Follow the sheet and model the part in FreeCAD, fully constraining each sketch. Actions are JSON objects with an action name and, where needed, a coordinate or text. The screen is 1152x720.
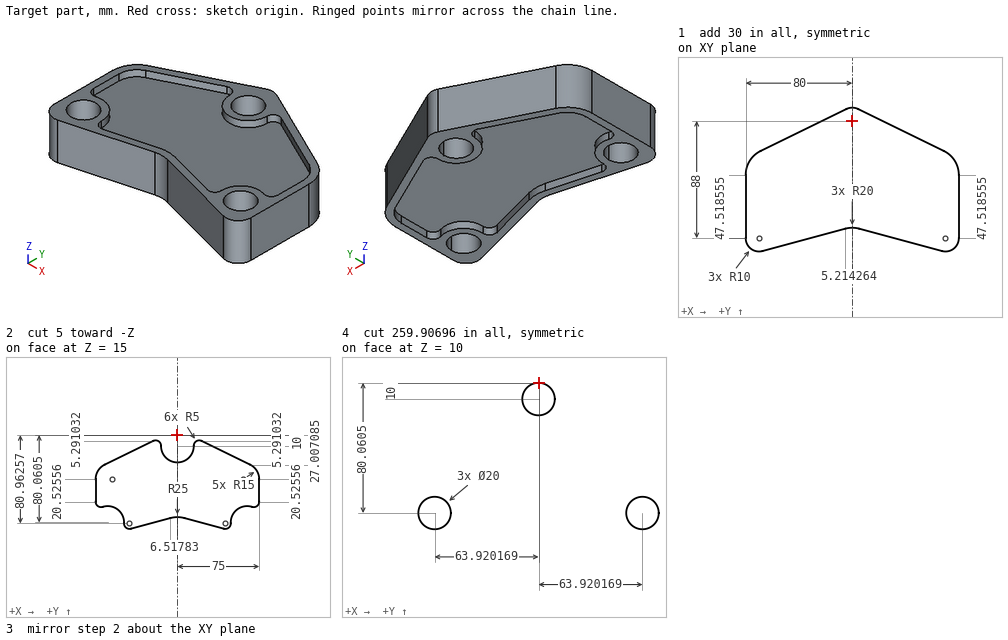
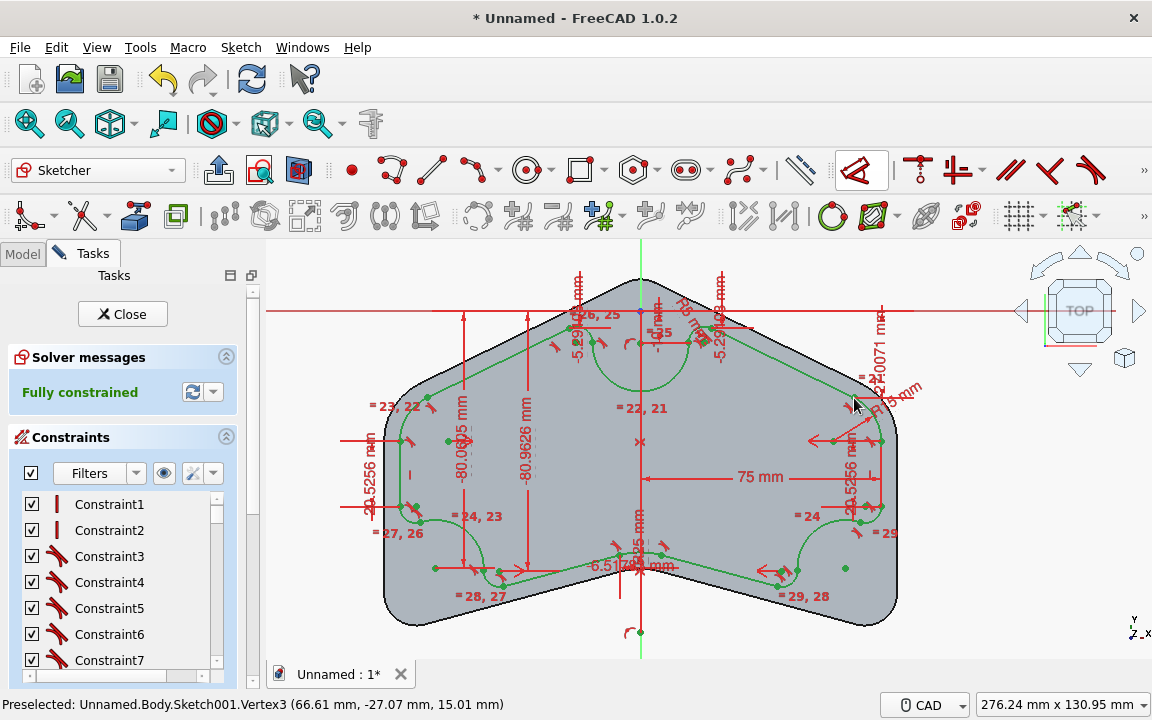
{"action": "left_click", "coordinate": [123, 314]}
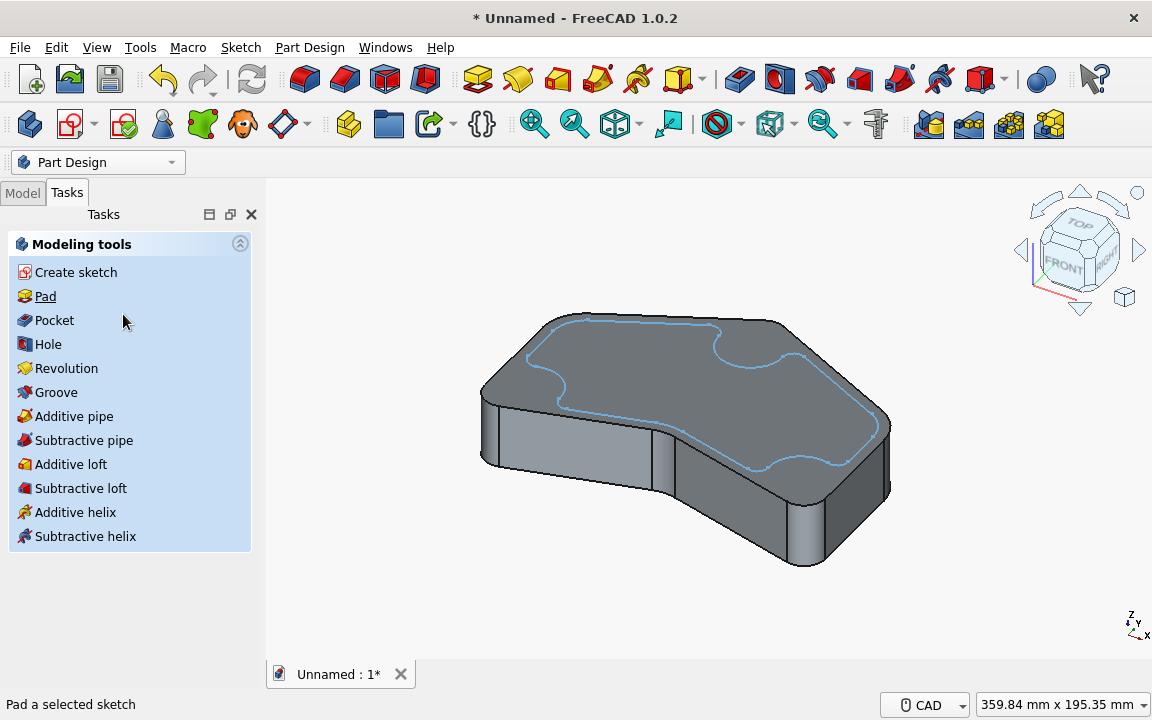
{"action": "left_click", "coordinate": [740, 80]}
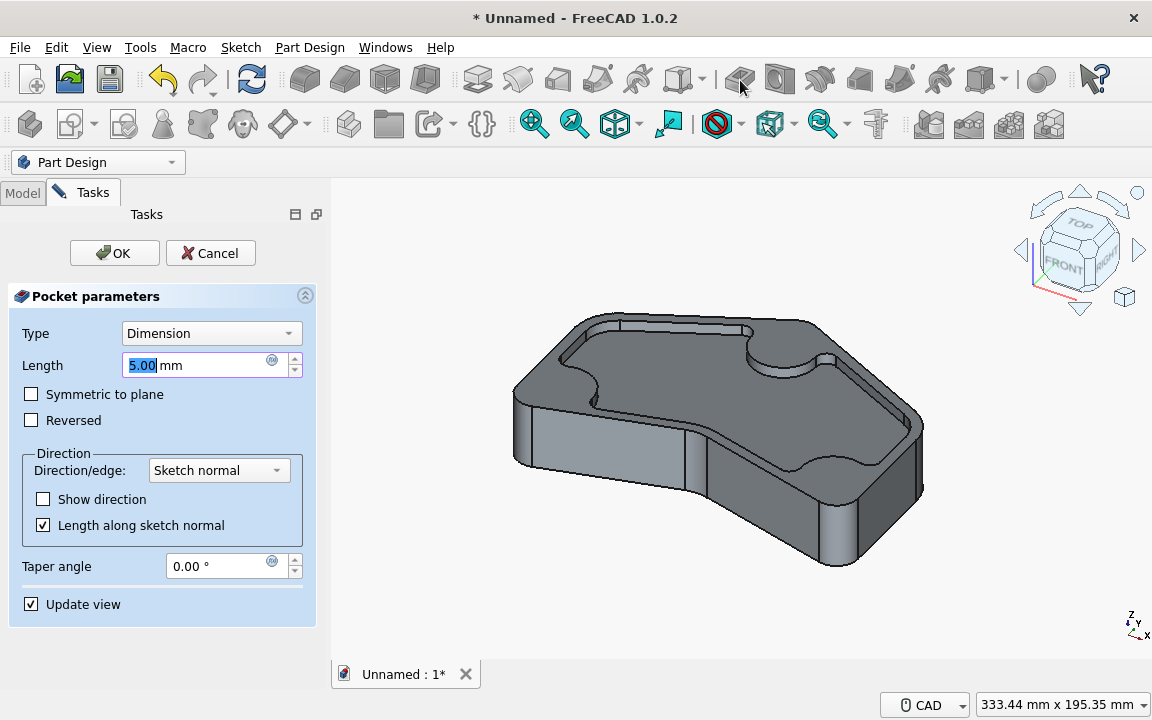
{"action": "type", "text": "5"}
{"action": "key", "text": "Tab"}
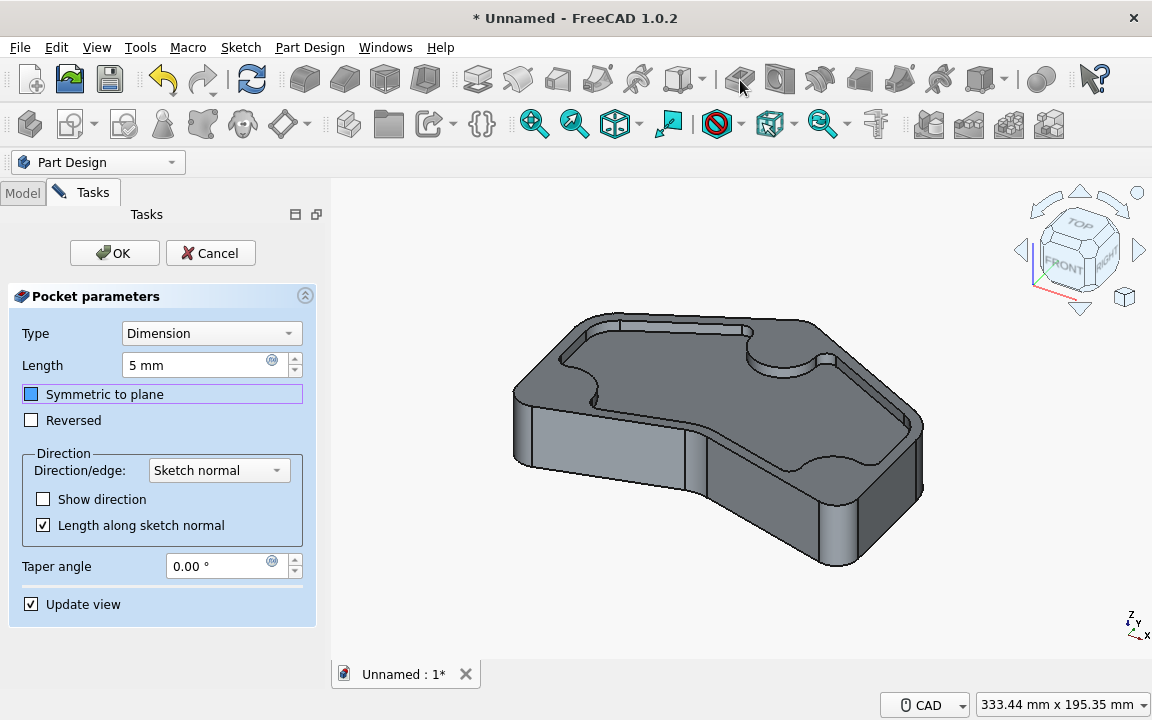
{"action": "left_click", "coordinate": [115, 253]}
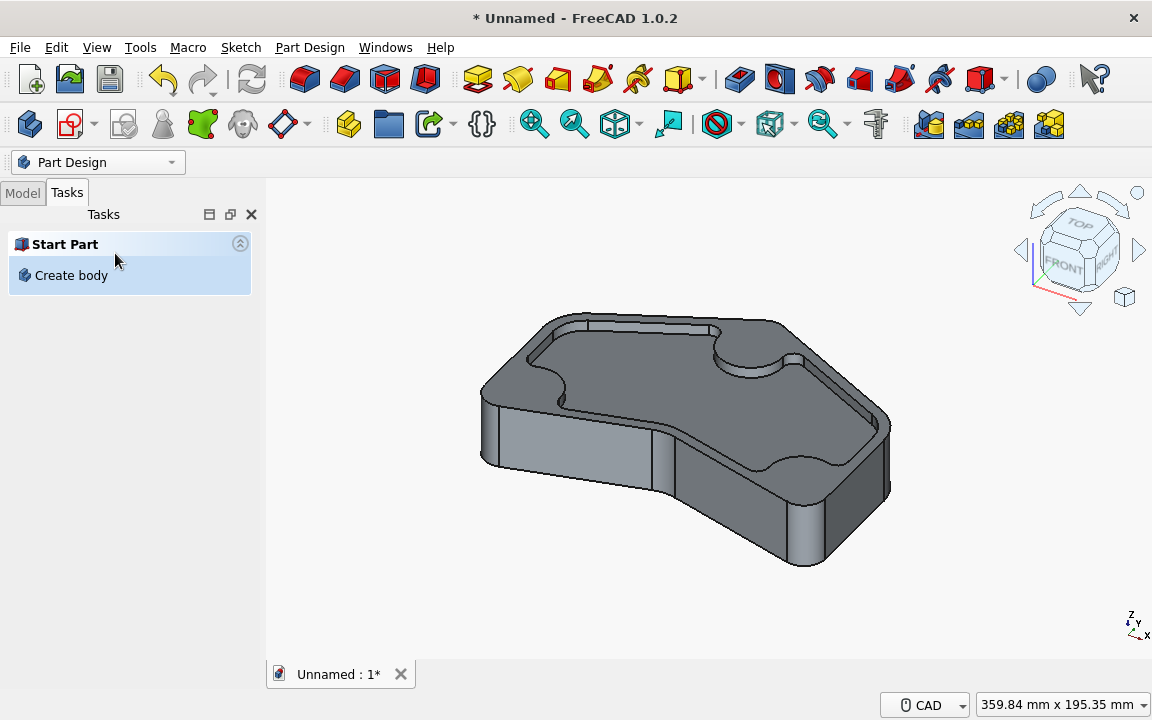
{"action": "left_click", "coordinate": [23, 192]}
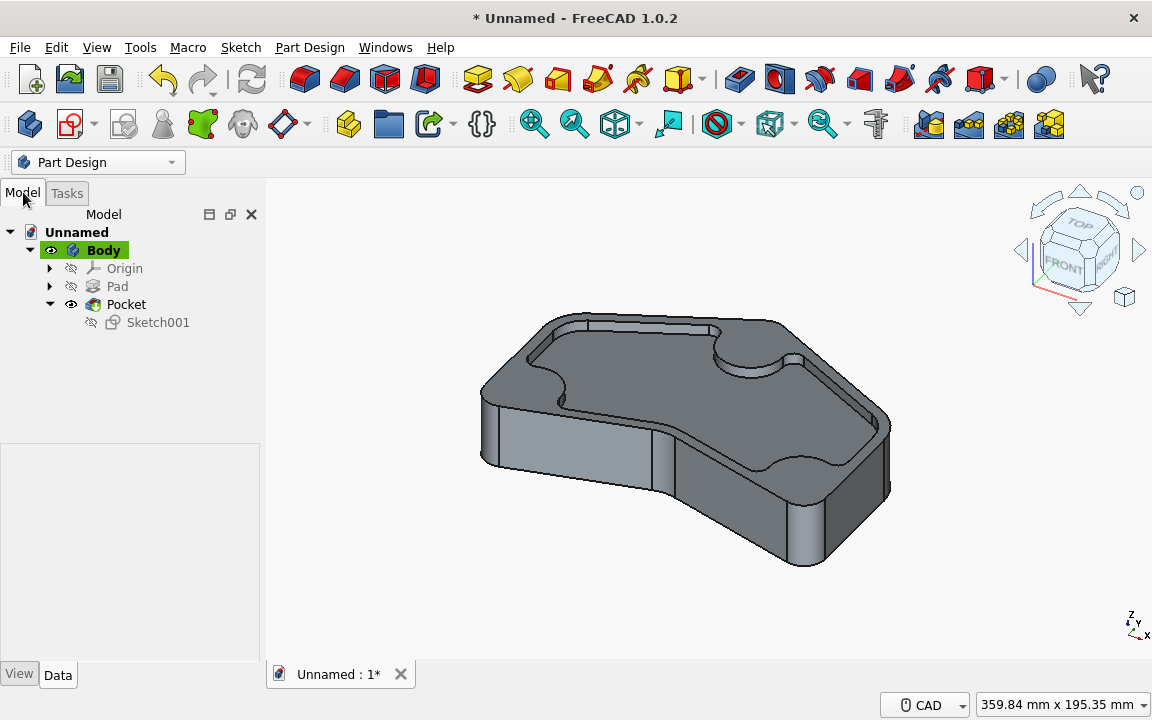
{"action": "left_click", "coordinate": [116, 304]}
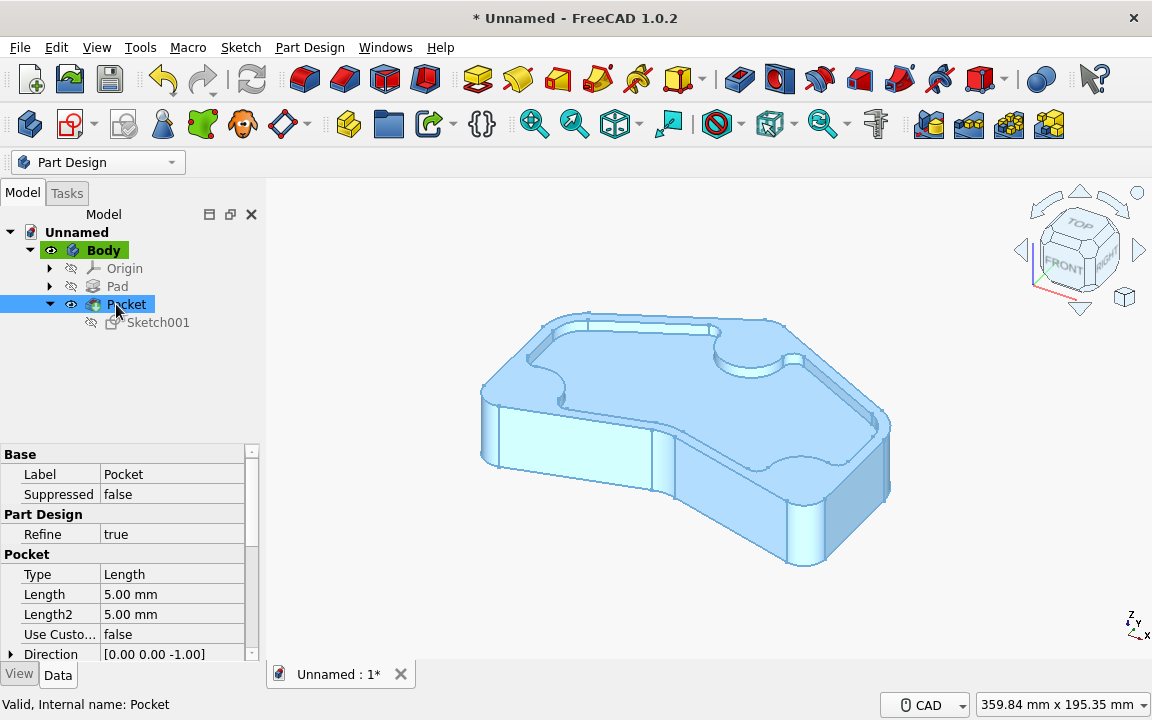
{"action": "left_click", "coordinate": [930, 124]}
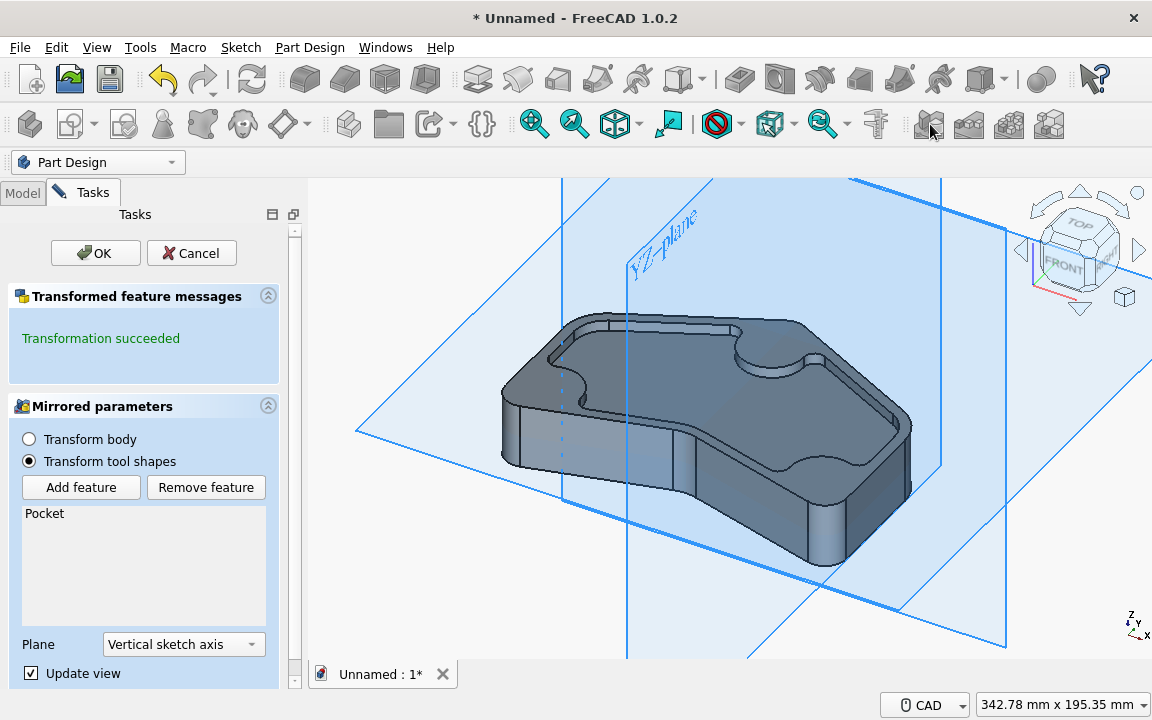
{"action": "left_click", "coordinate": [184, 644]}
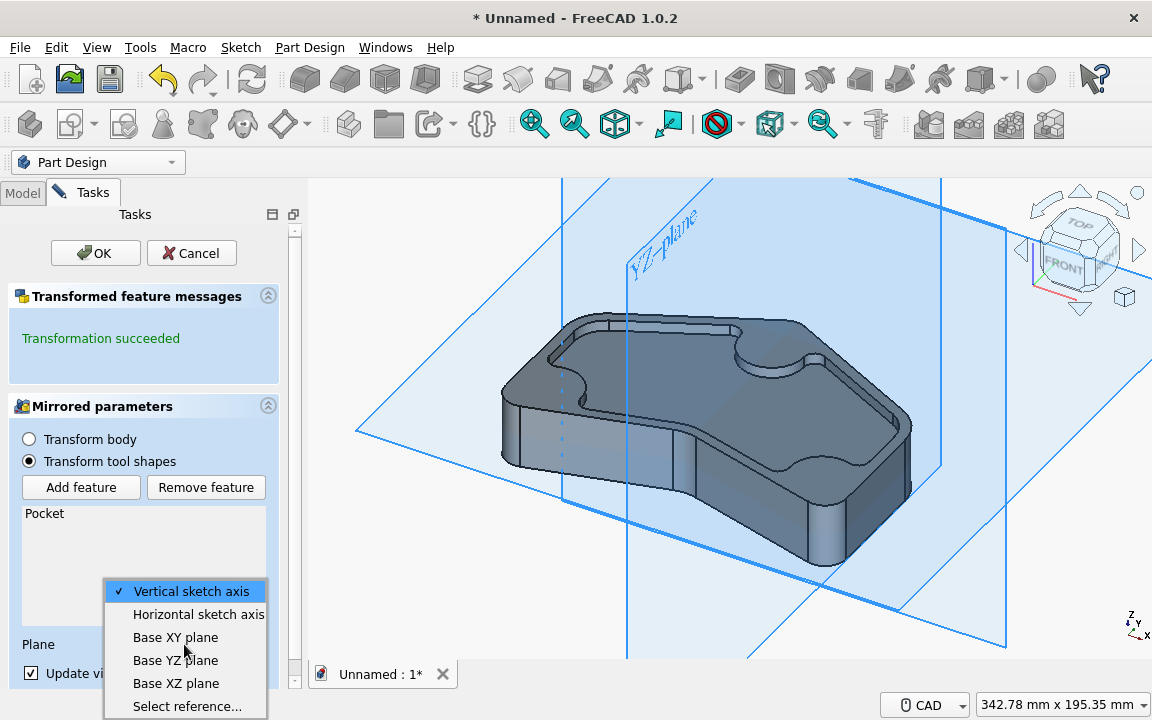
{"action": "left_click", "coordinate": [184, 638]}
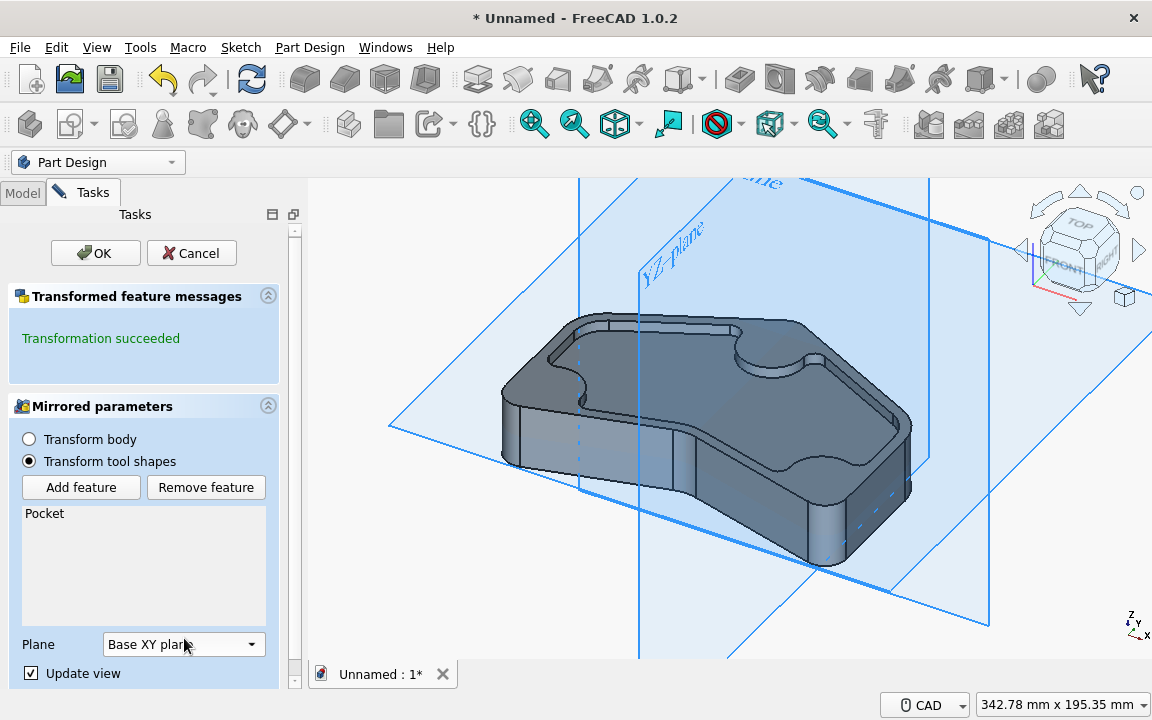
{"action": "left_click", "coordinate": [96, 253]}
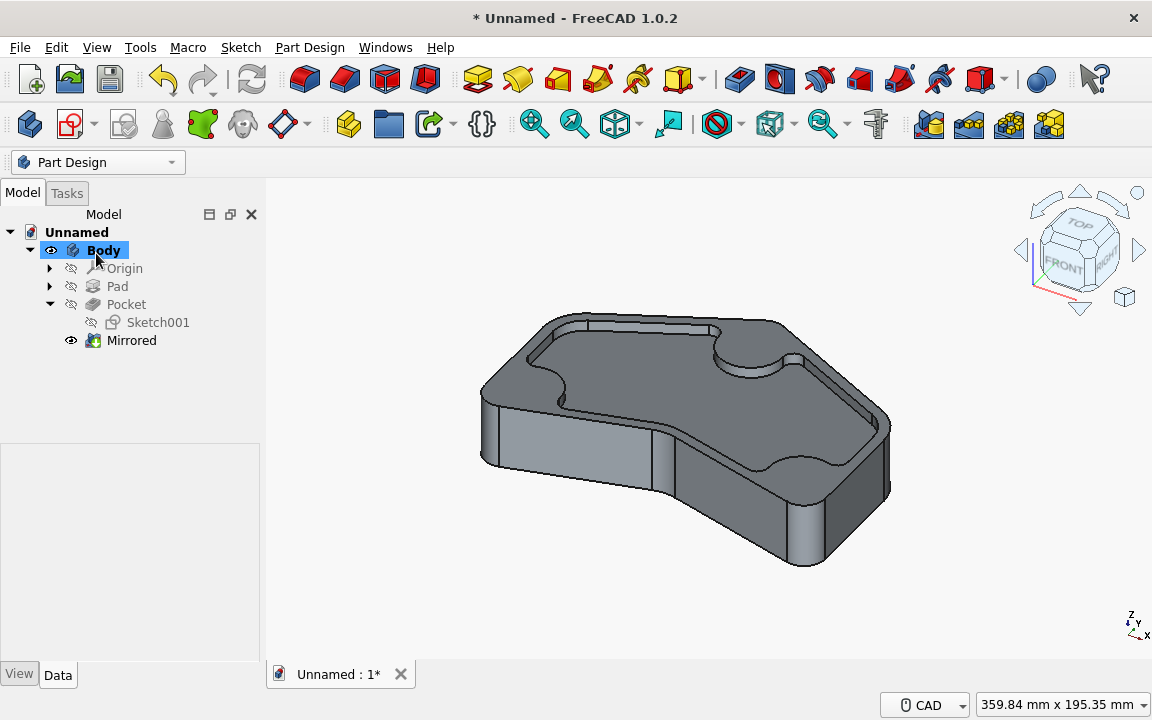
{"action": "left_click", "coordinate": [662, 384]}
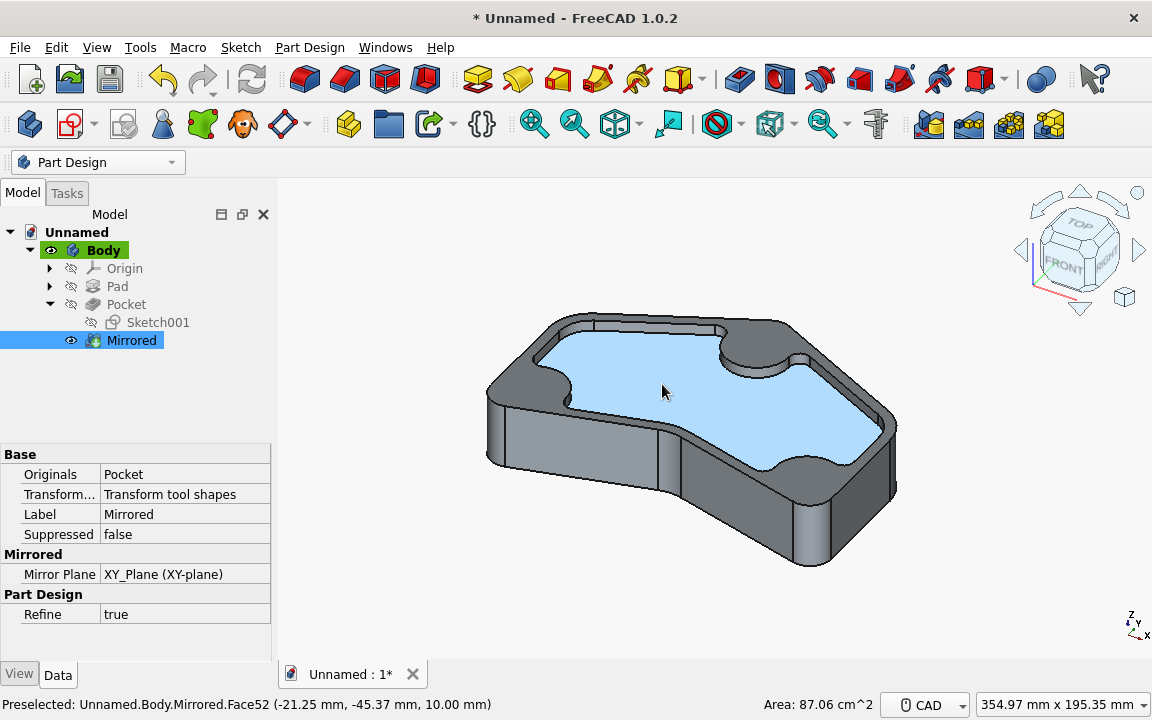
{"action": "left_click", "coordinate": [70, 124]}